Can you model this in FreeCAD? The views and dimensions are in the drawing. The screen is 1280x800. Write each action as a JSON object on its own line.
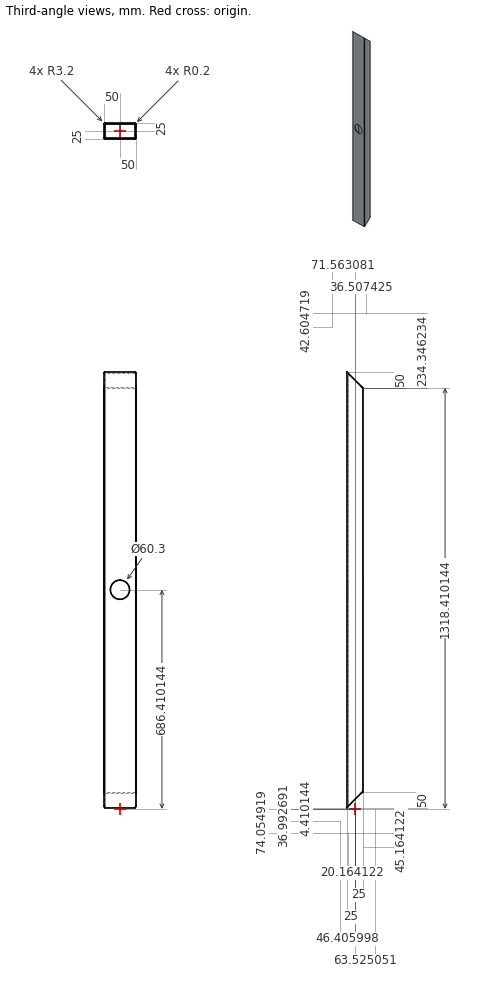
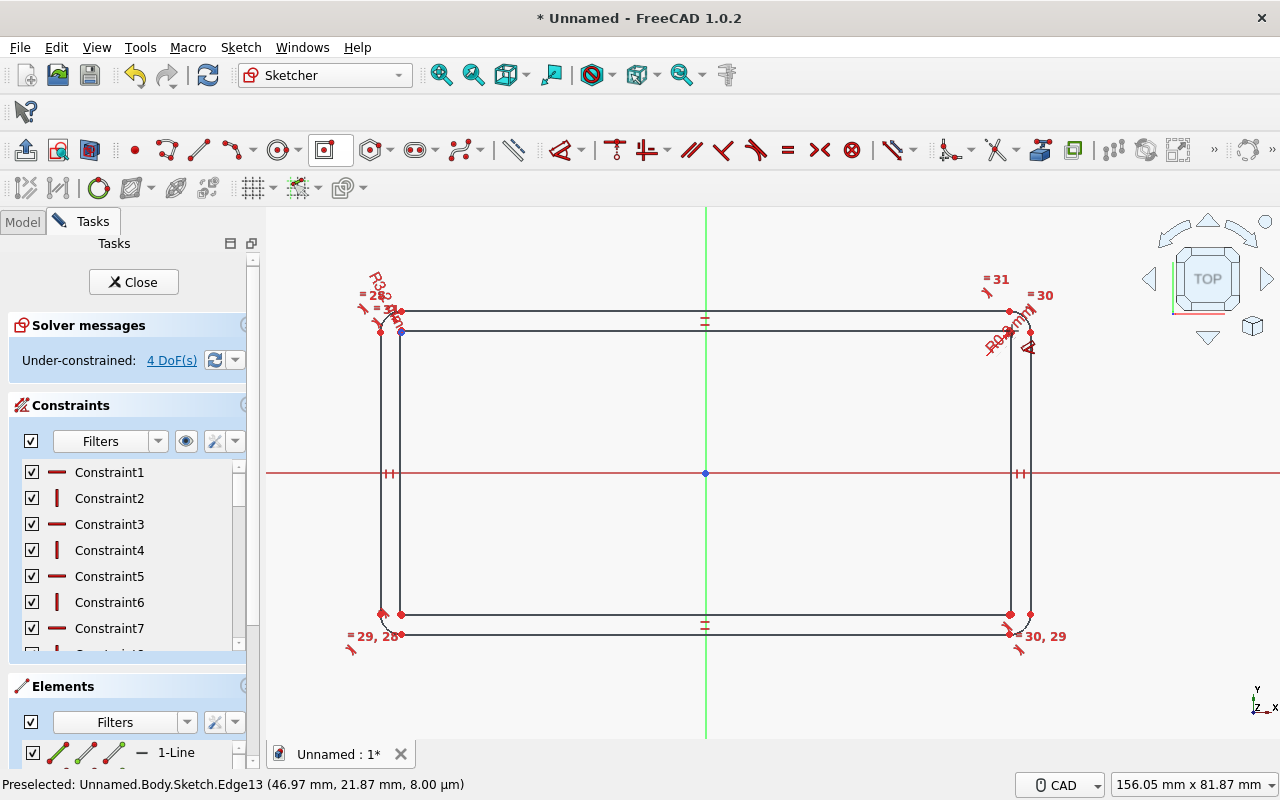
{"action": "left_click", "coordinate": [1010, 311]}
{"action": "left_click", "coordinate": [1044, 392]}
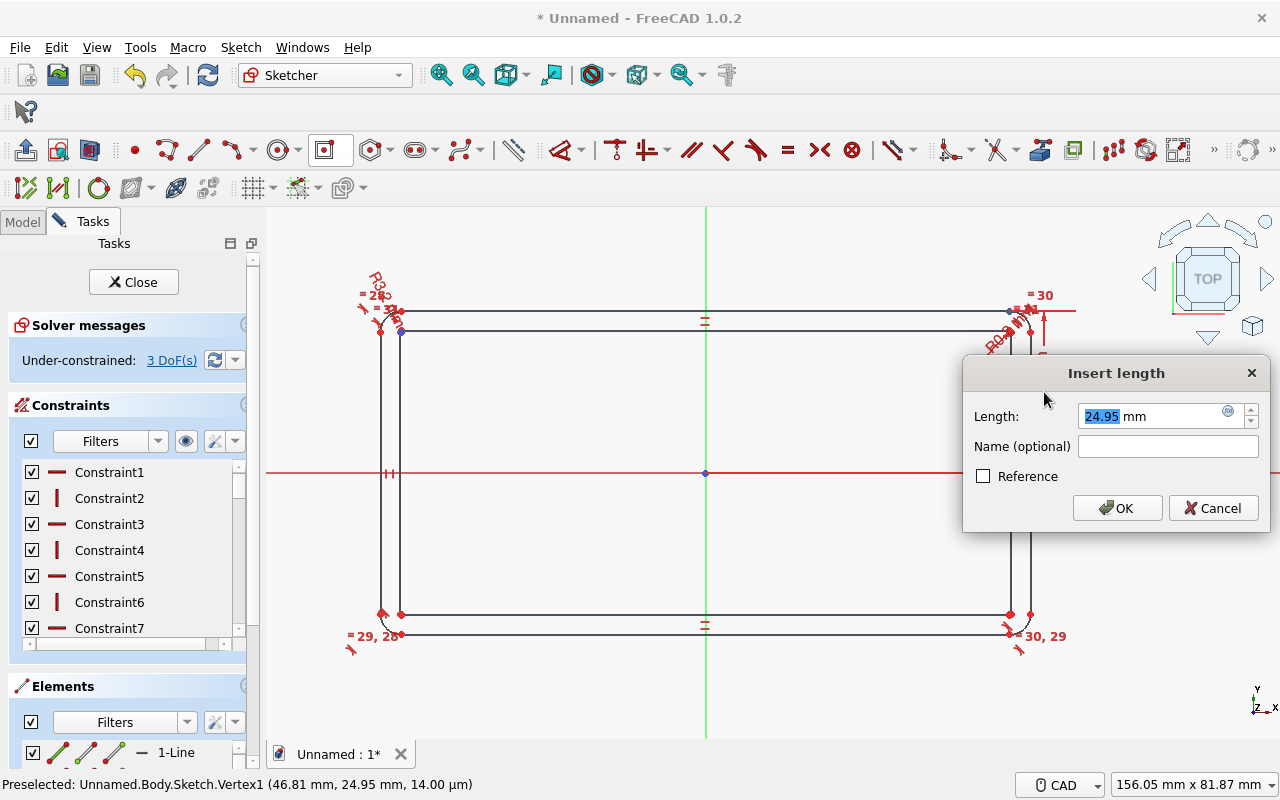
{"action": "type", "text": "25"}
{"action": "key", "text": "Return"}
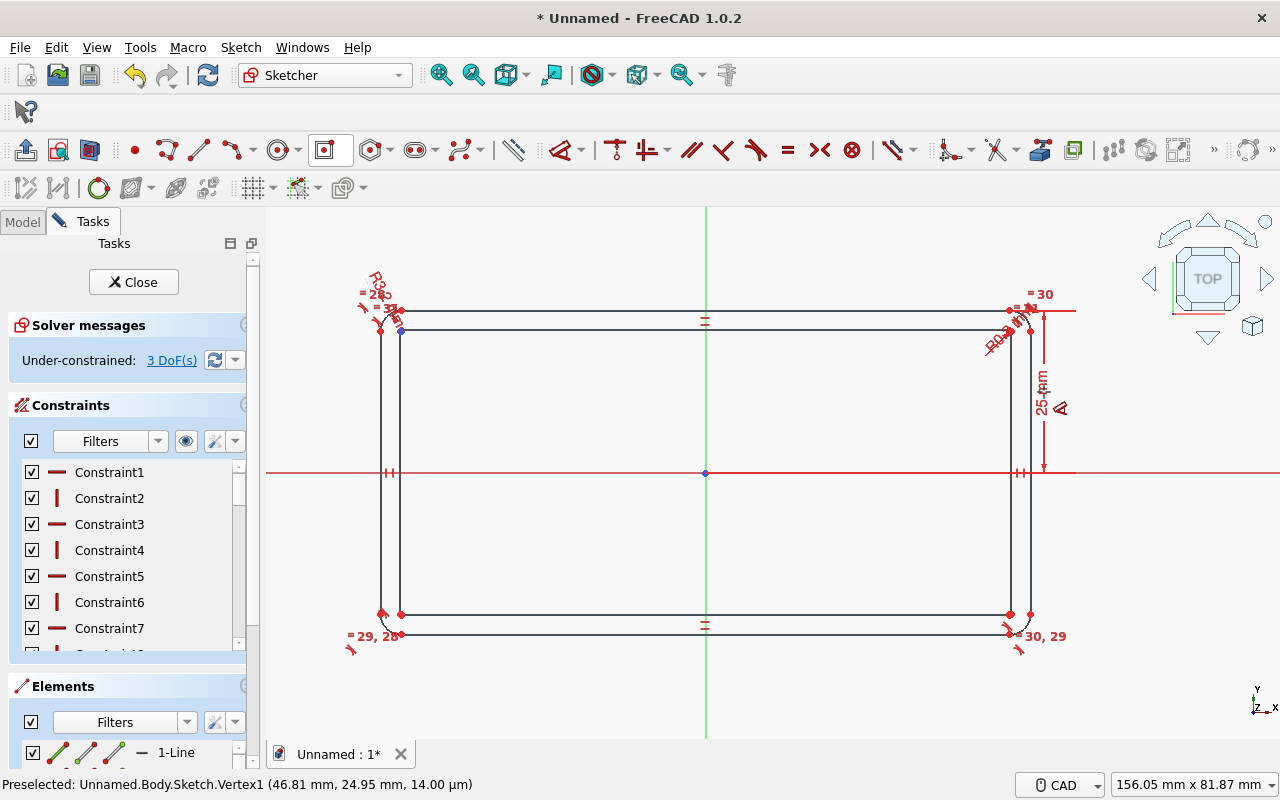
{"action": "left_click", "coordinate": [381, 332]}
{"action": "left_click", "coordinate": [543, 298]}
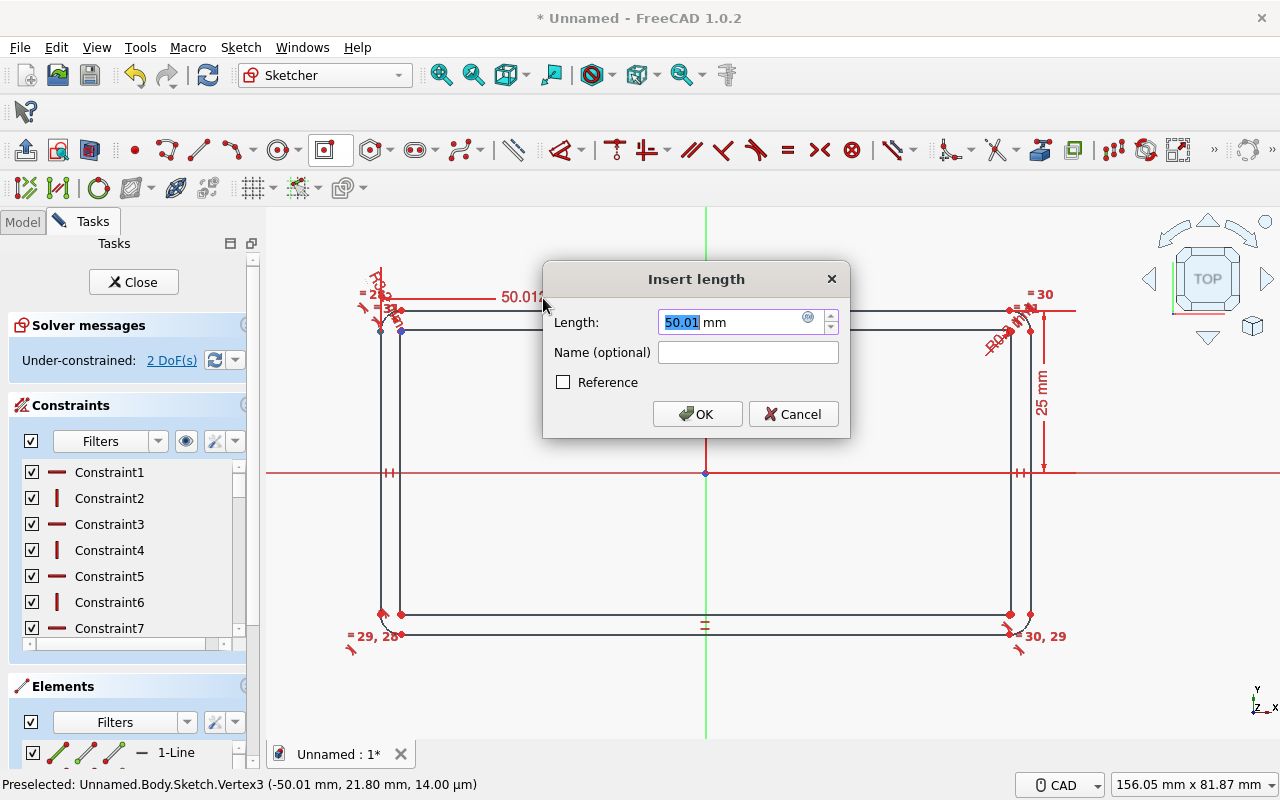
{"action": "type", "text": "50"}
{"action": "key", "text": "Return"}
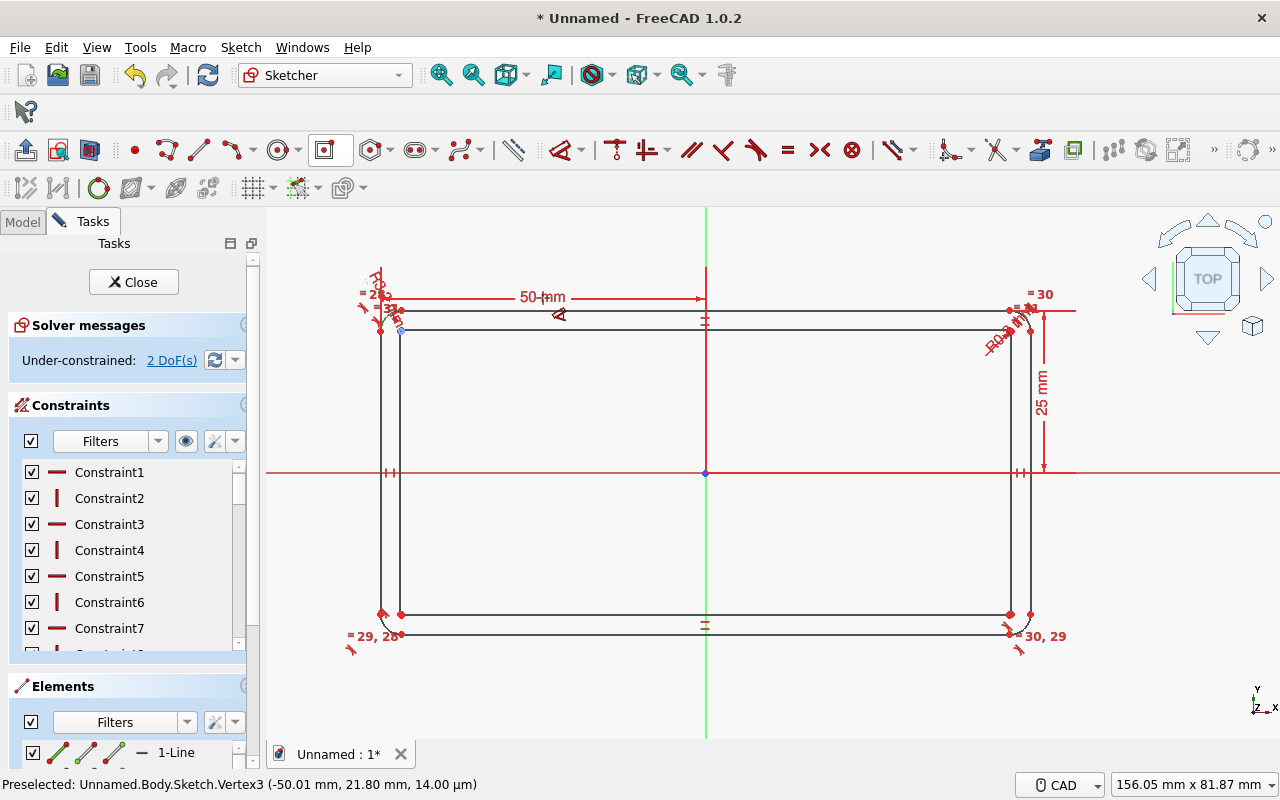
{"action": "left_click", "coordinate": [402, 635]}
{"action": "left_click", "coordinate": [368, 554]}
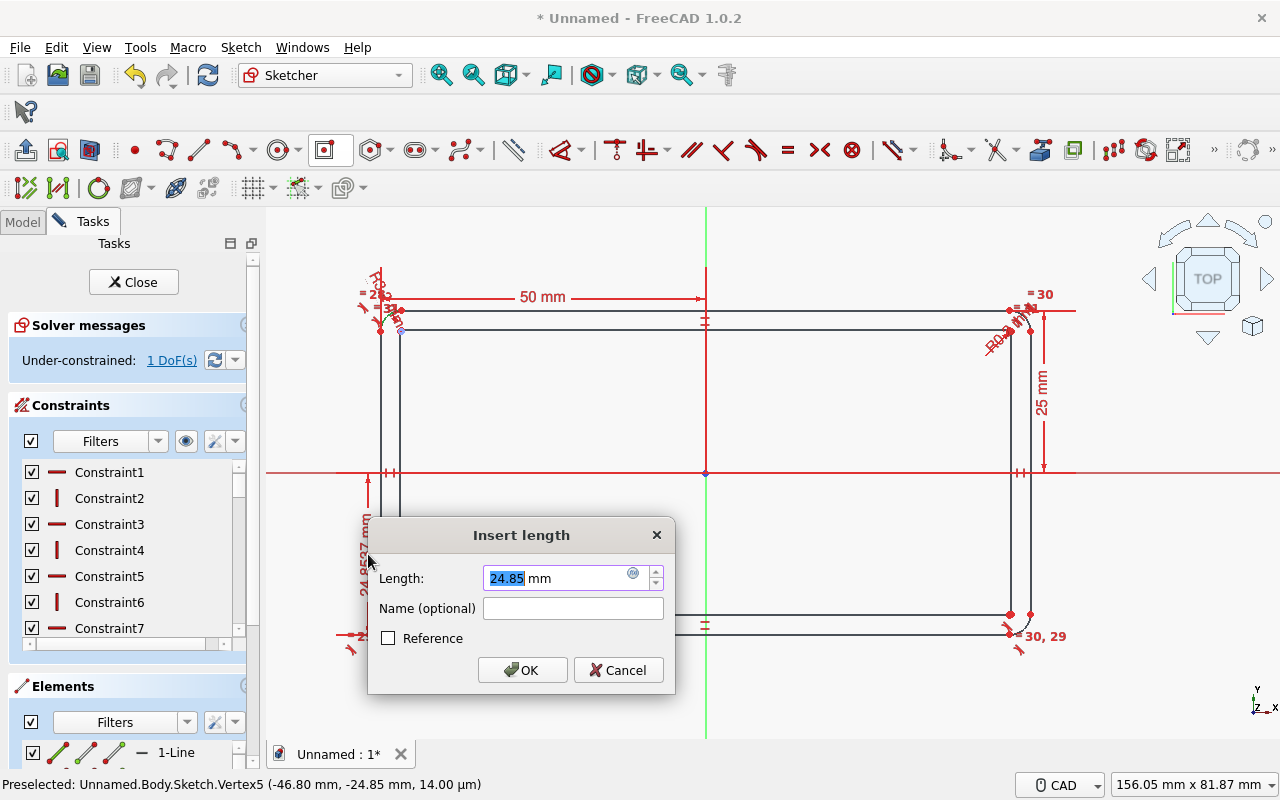
{"action": "type", "text": "25"}
{"action": "key", "text": "Return"}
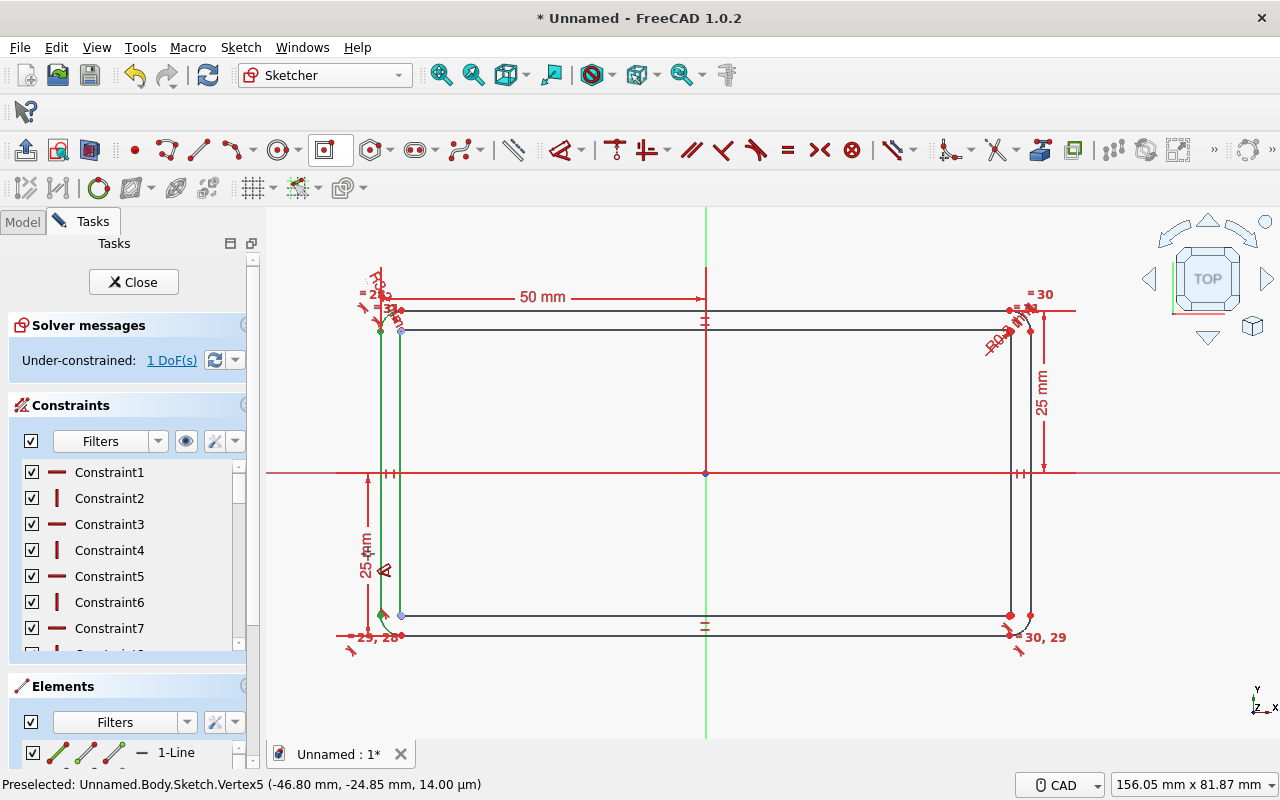
{"action": "left_click", "coordinate": [1031, 615]}
{"action": "left_click", "coordinate": [868, 649]}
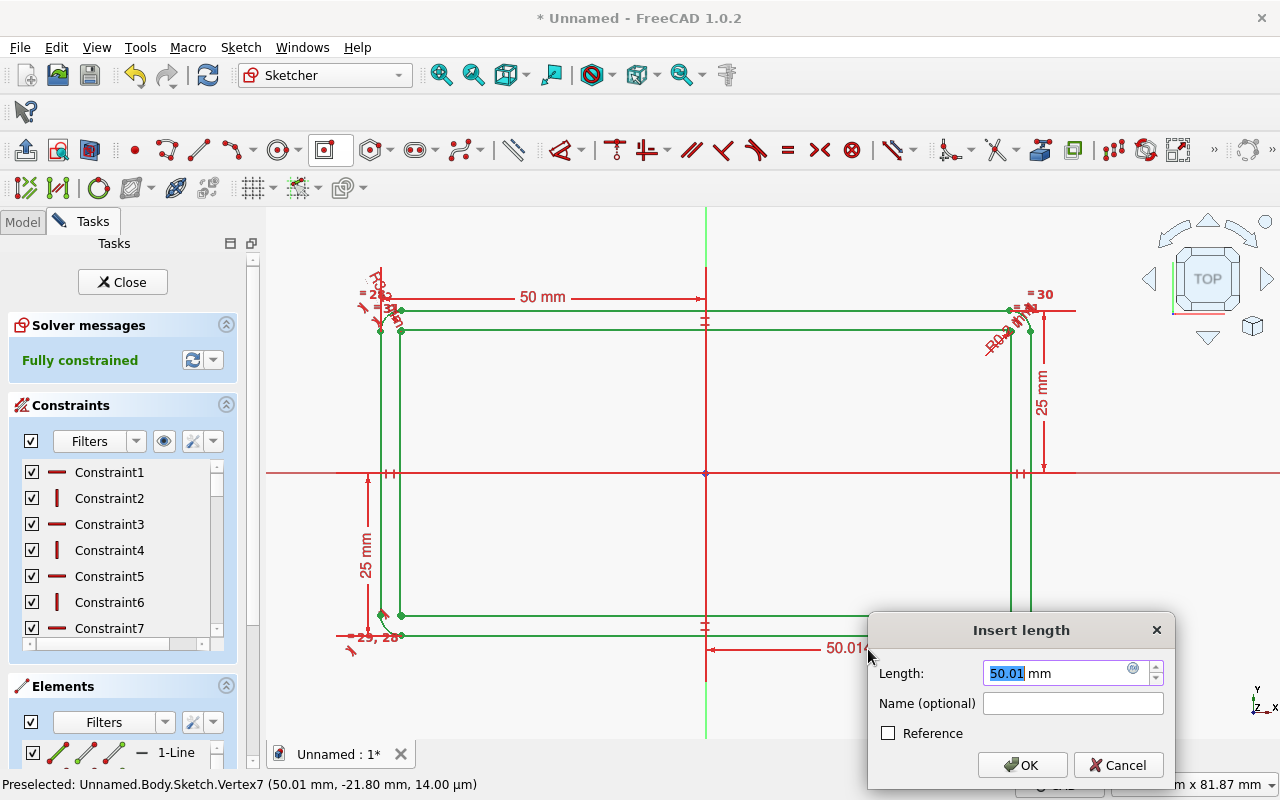
{"action": "type", "text": "50"}
{"action": "key", "text": "Return"}
{"action": "key", "text": "Escape"}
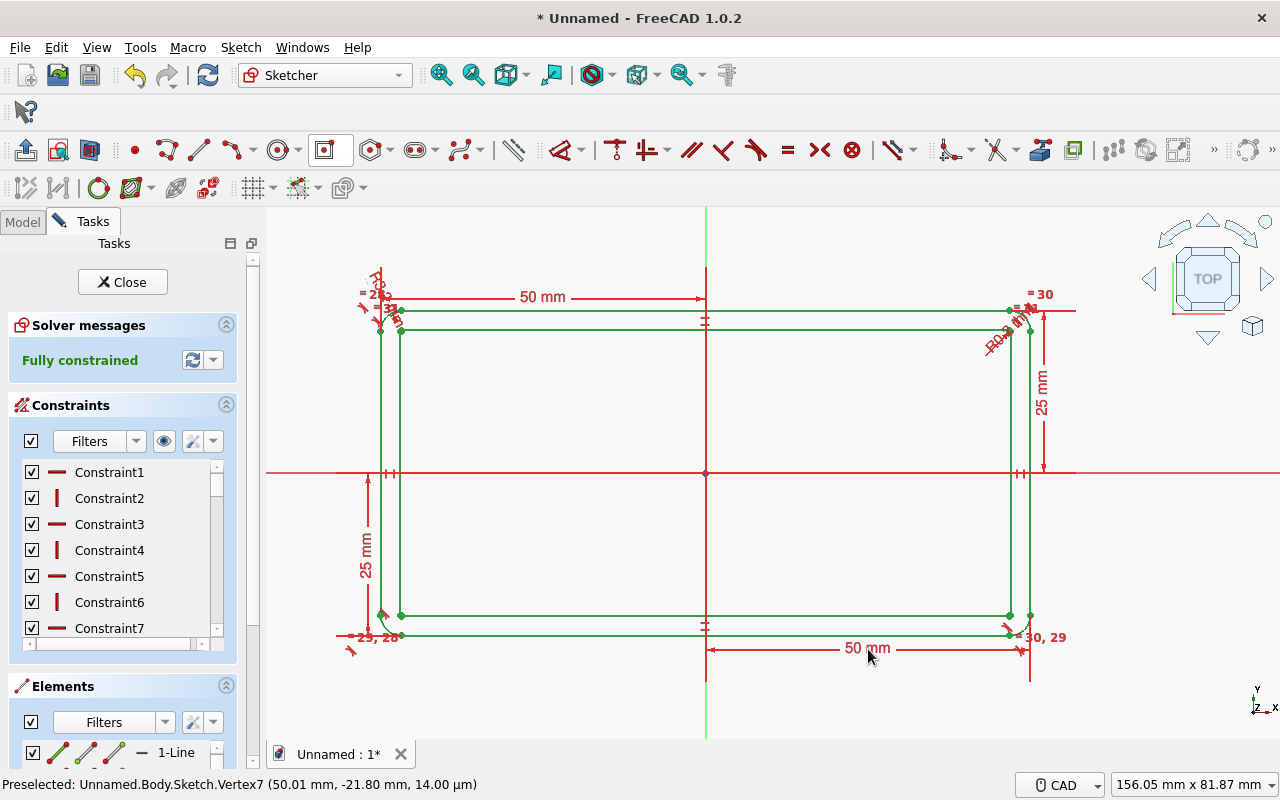
{"action": "left_click", "coordinate": [123, 282]}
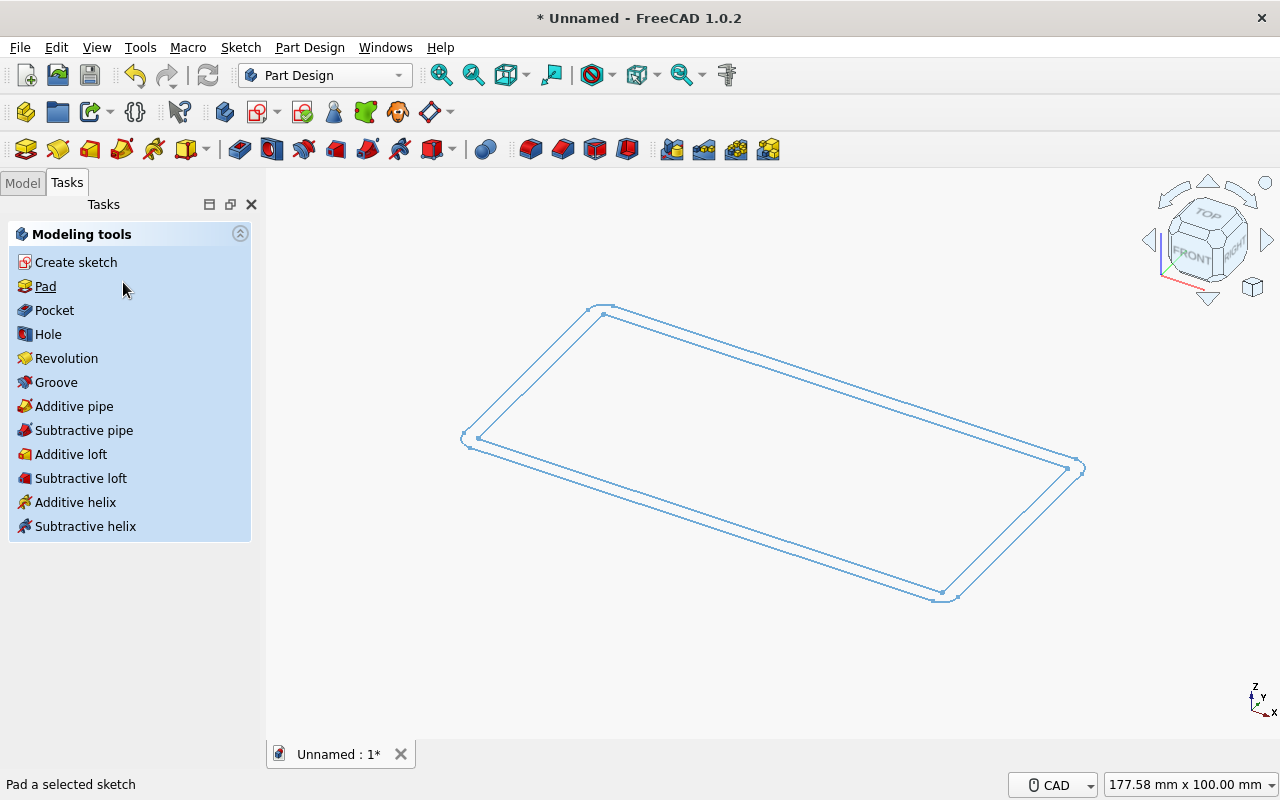
{"action": "left_click", "coordinate": [26, 150]}